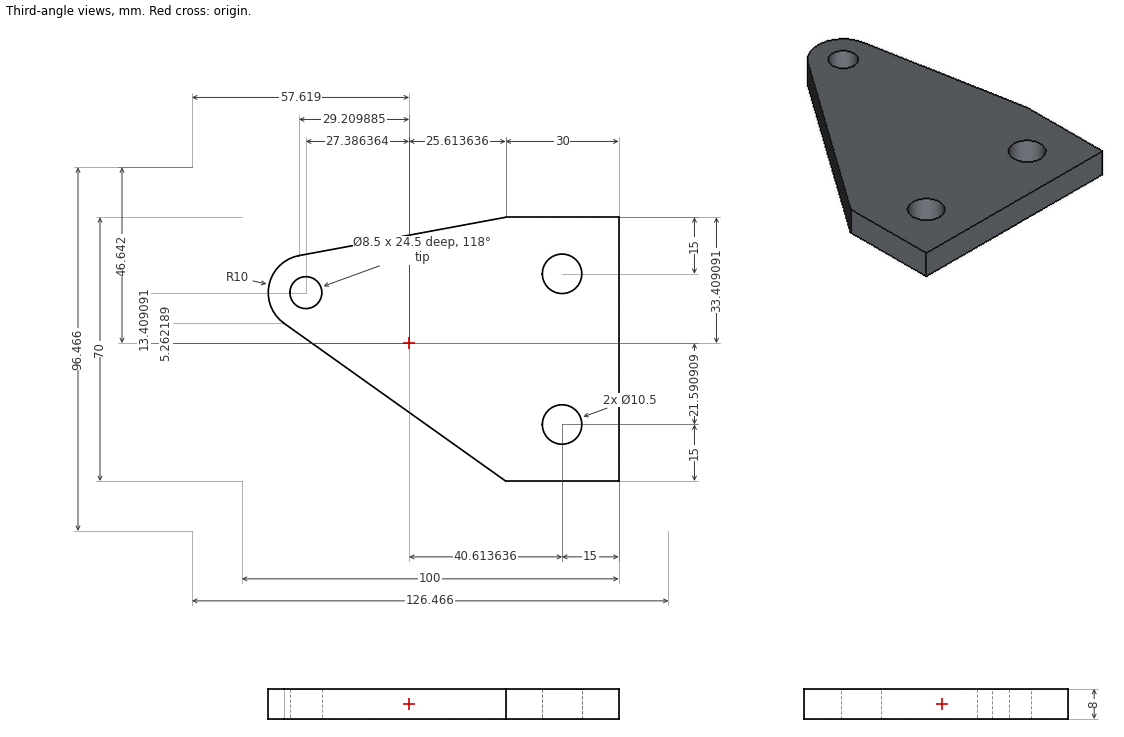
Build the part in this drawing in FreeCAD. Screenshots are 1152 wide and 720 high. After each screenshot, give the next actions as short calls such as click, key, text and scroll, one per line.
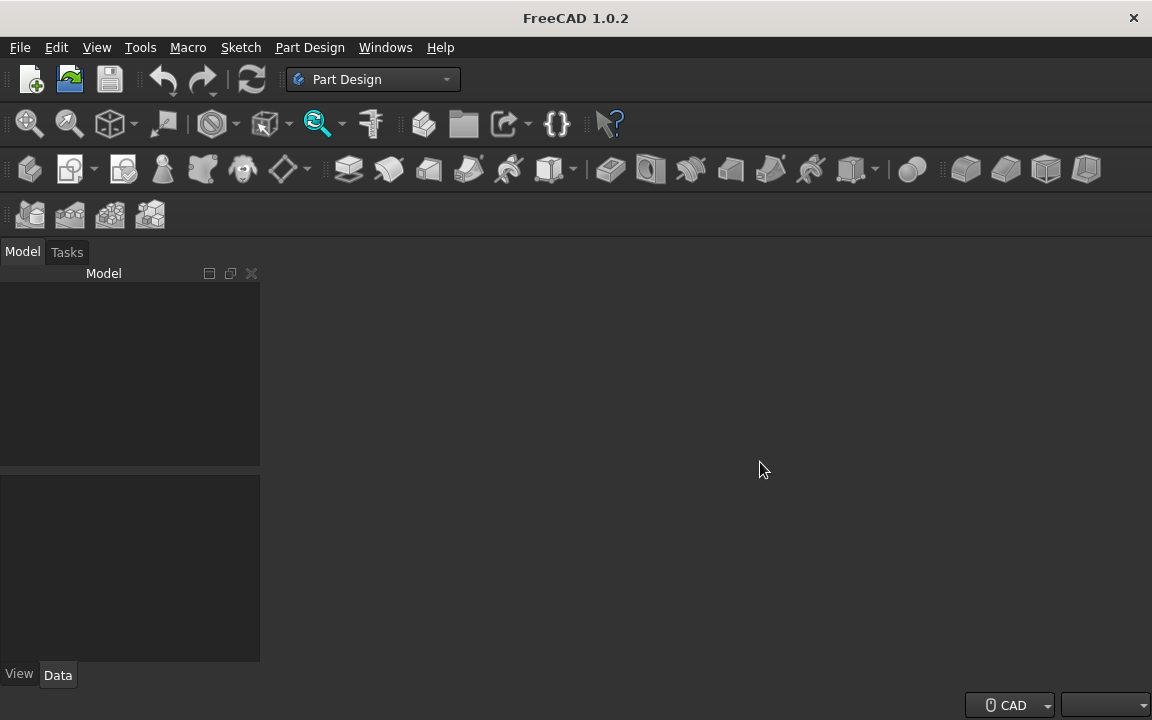
key(ctrl+n)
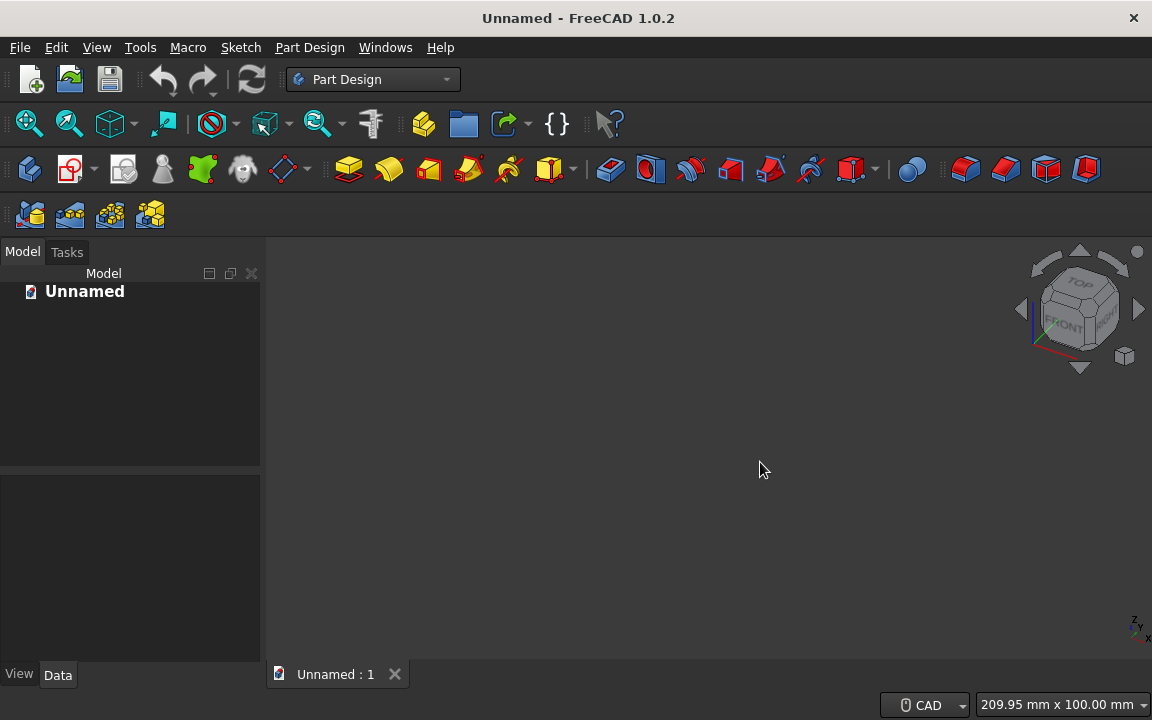
click(30, 170)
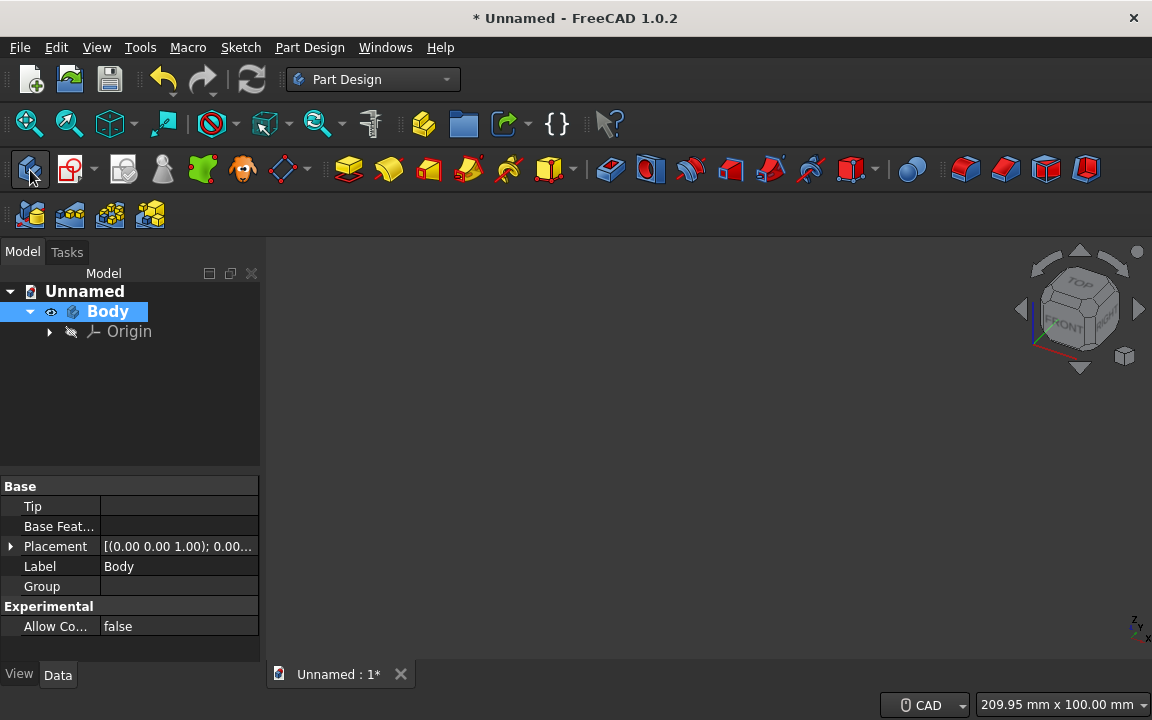
click(50, 332)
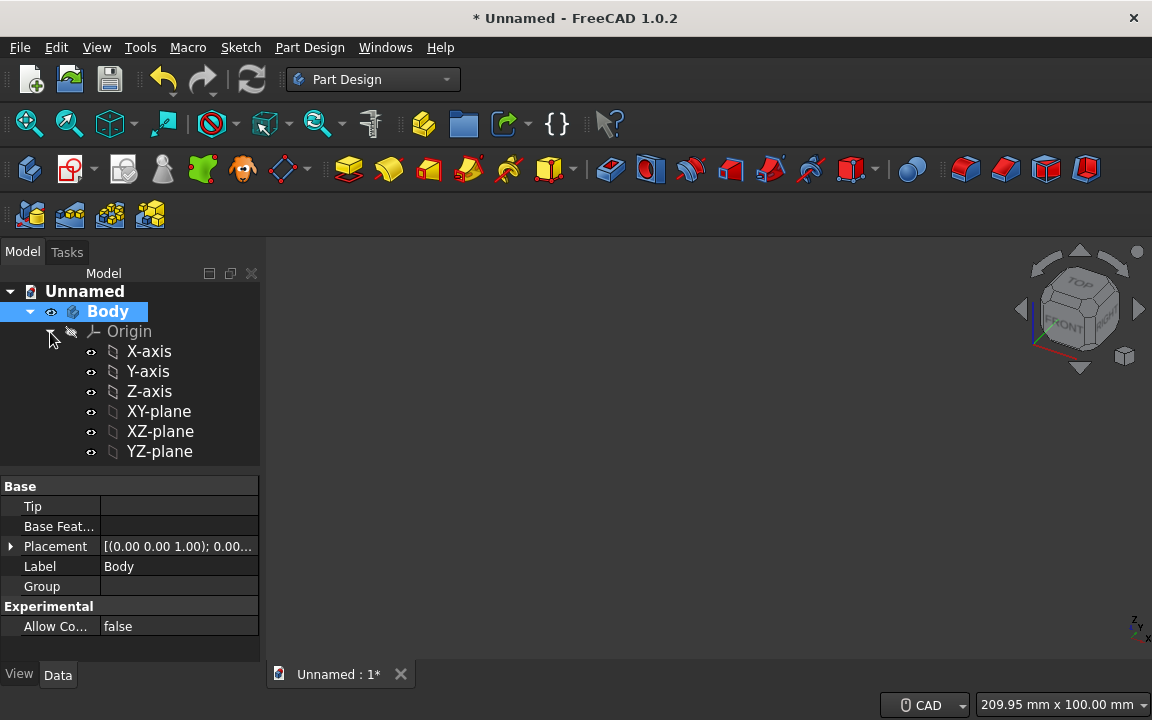
click(136, 412)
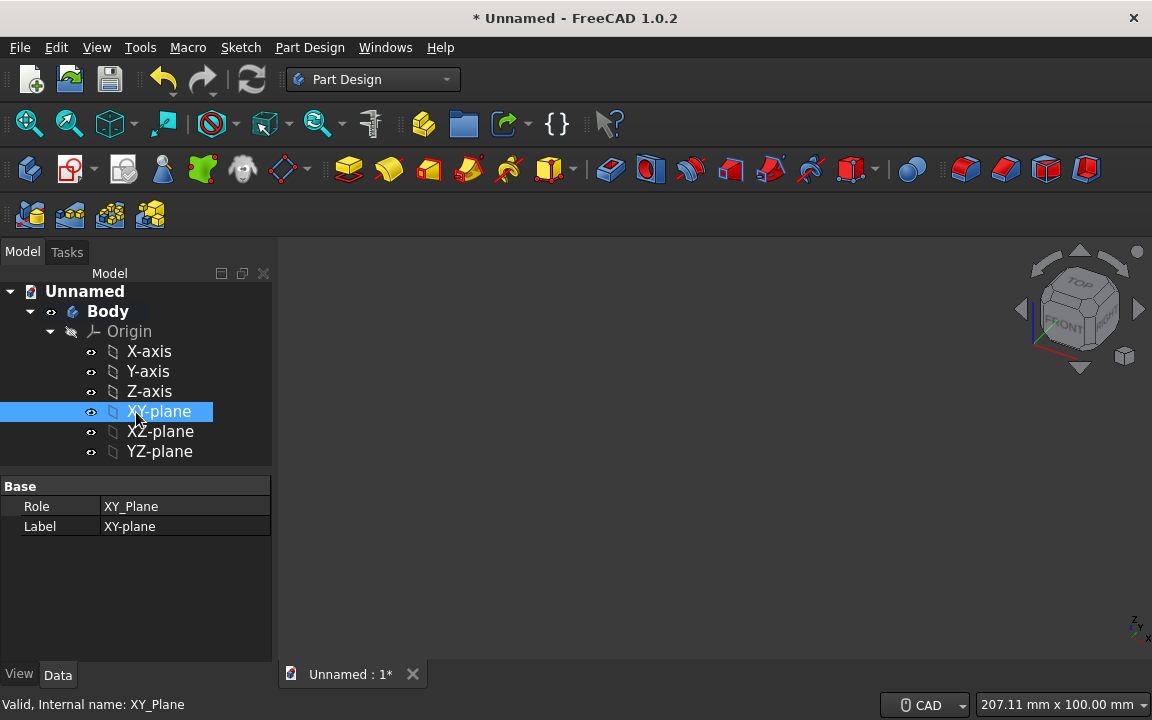
click(284, 170)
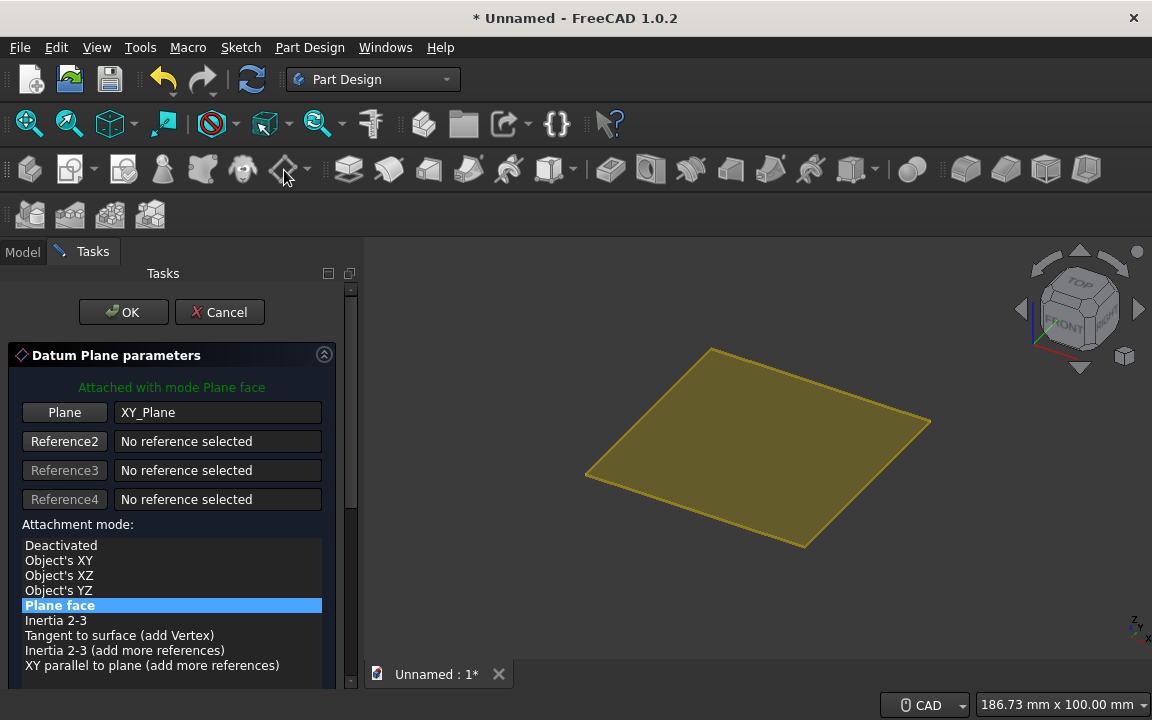
scroll(351, 486, down, 4)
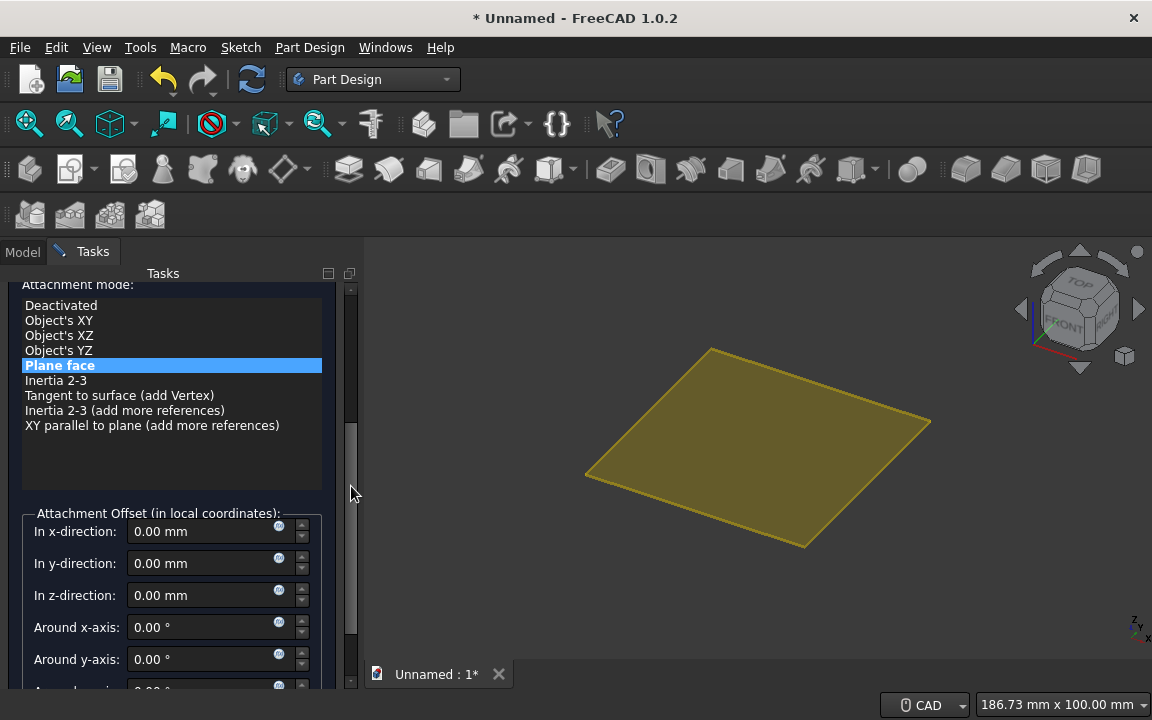
triple_click(210, 595)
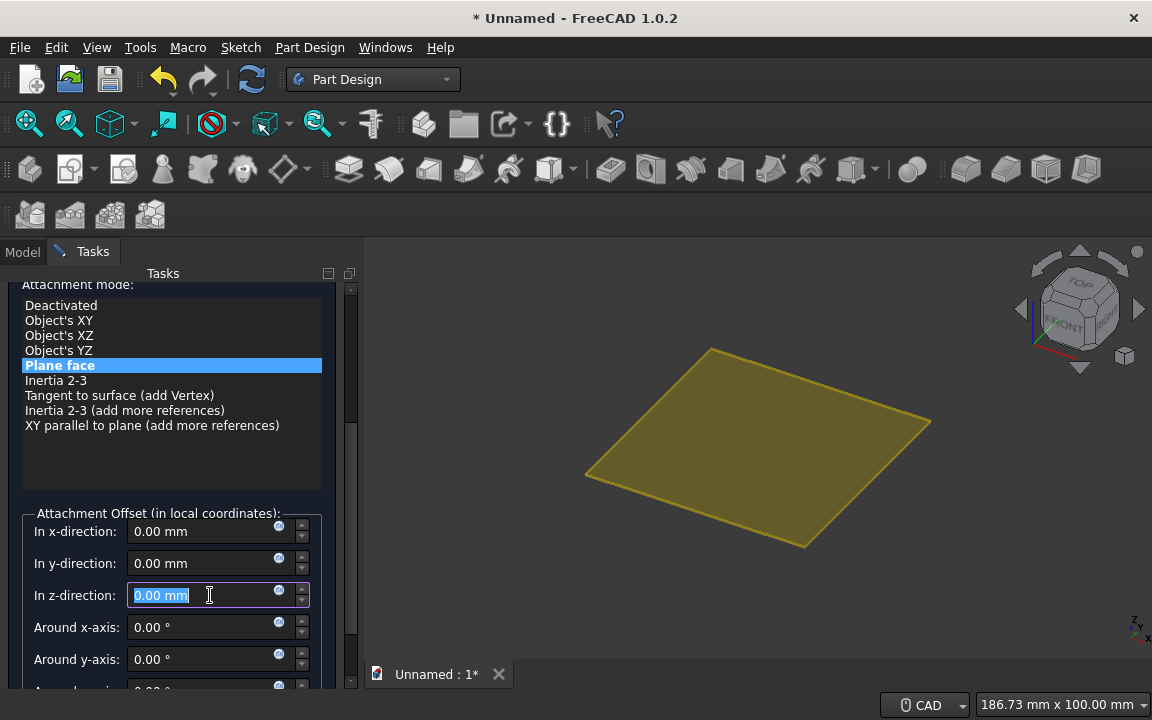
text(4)
key(Tab)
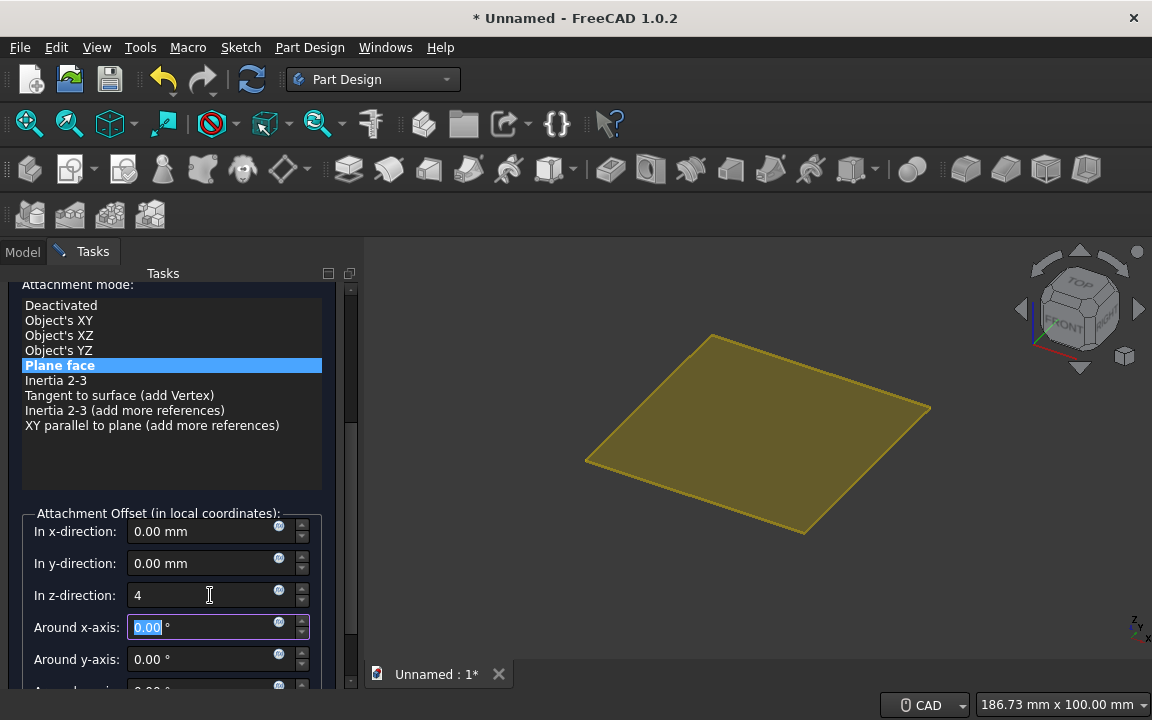
scroll(351, 486, up, 5)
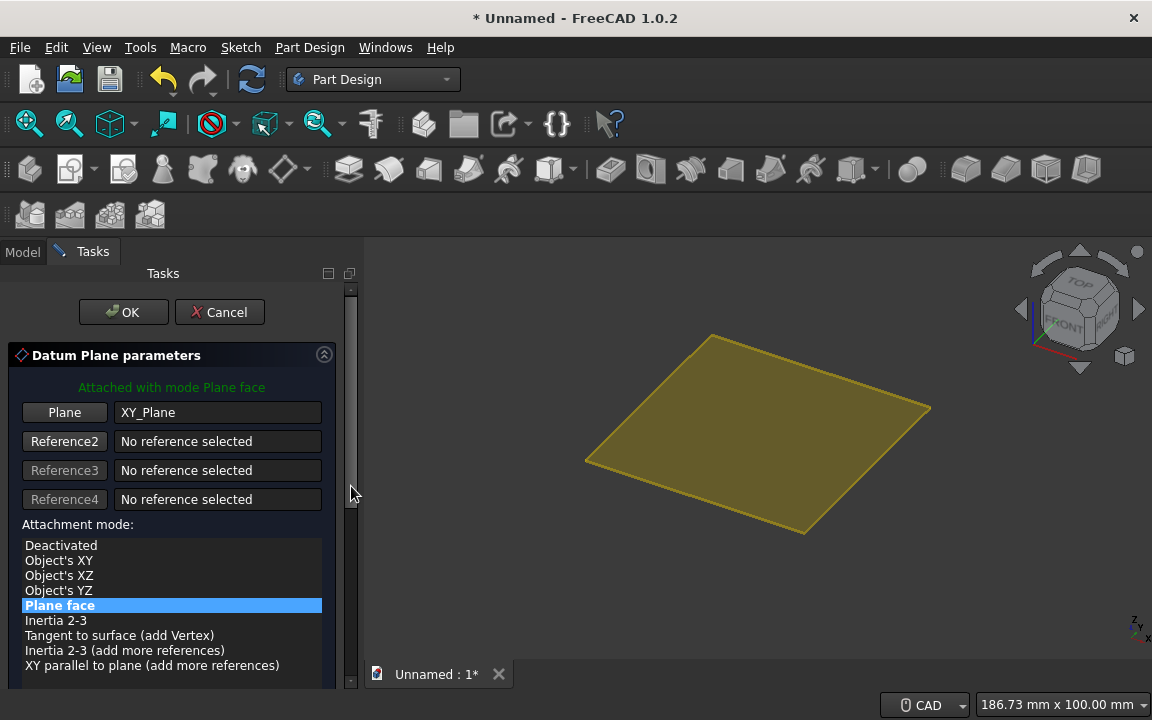
click(124, 312)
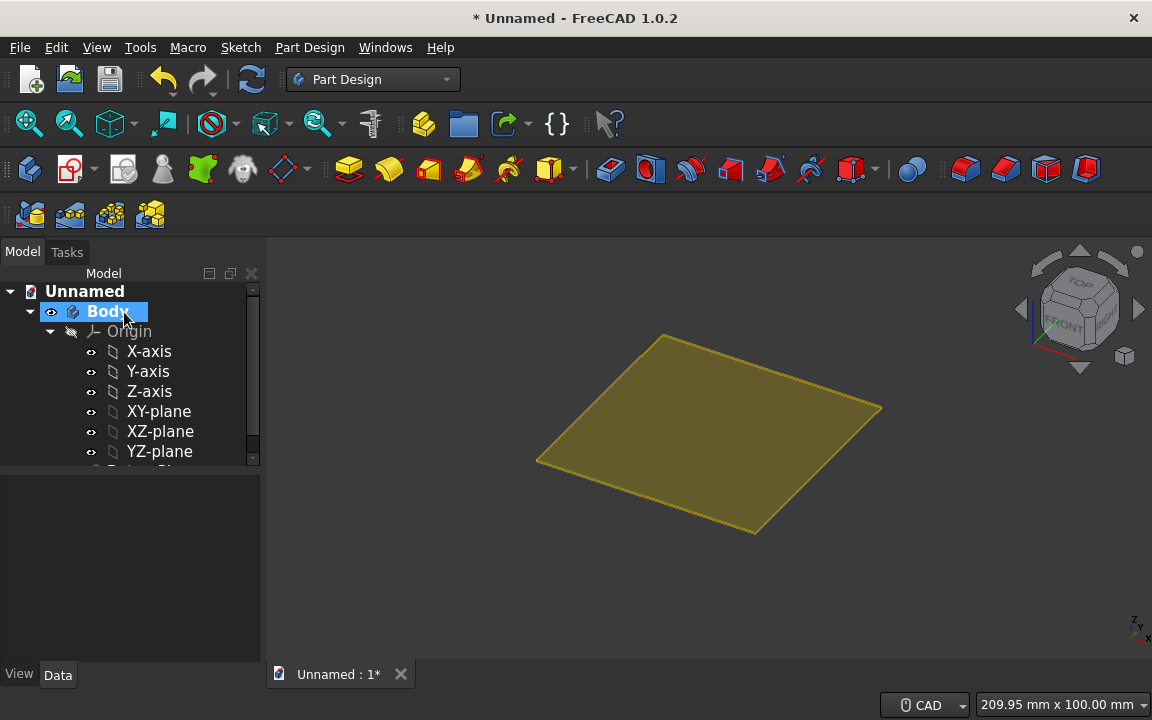
scroll(100, 367, down, 3)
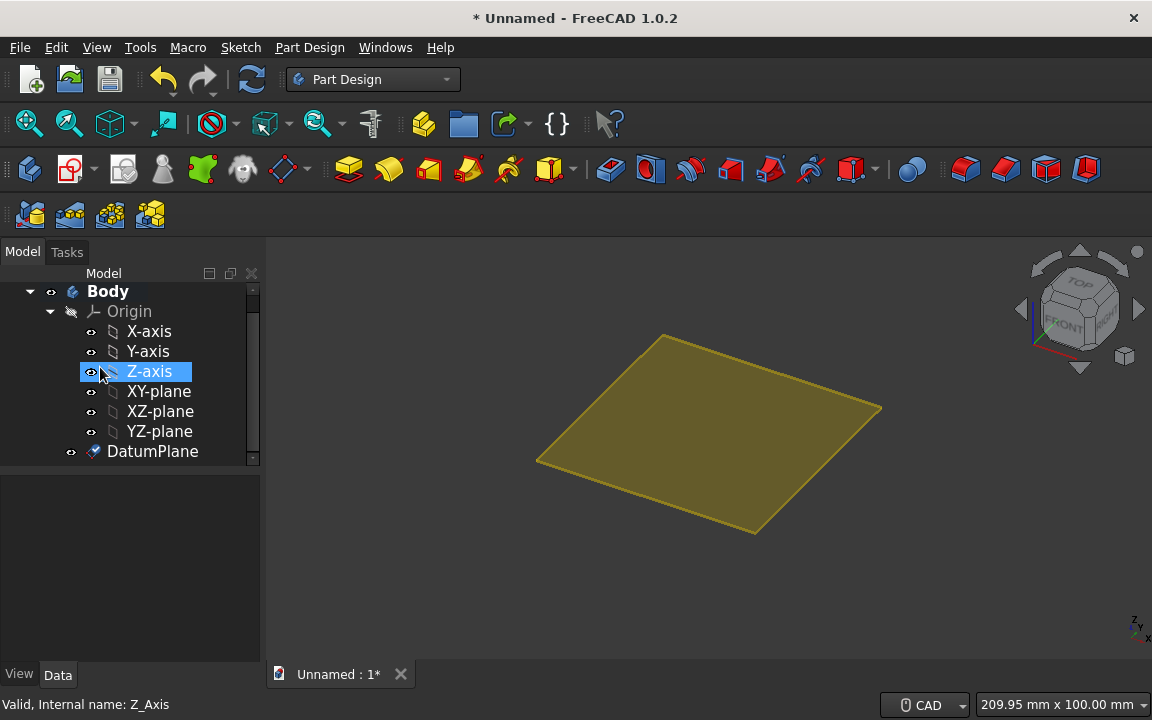
click(116, 452)